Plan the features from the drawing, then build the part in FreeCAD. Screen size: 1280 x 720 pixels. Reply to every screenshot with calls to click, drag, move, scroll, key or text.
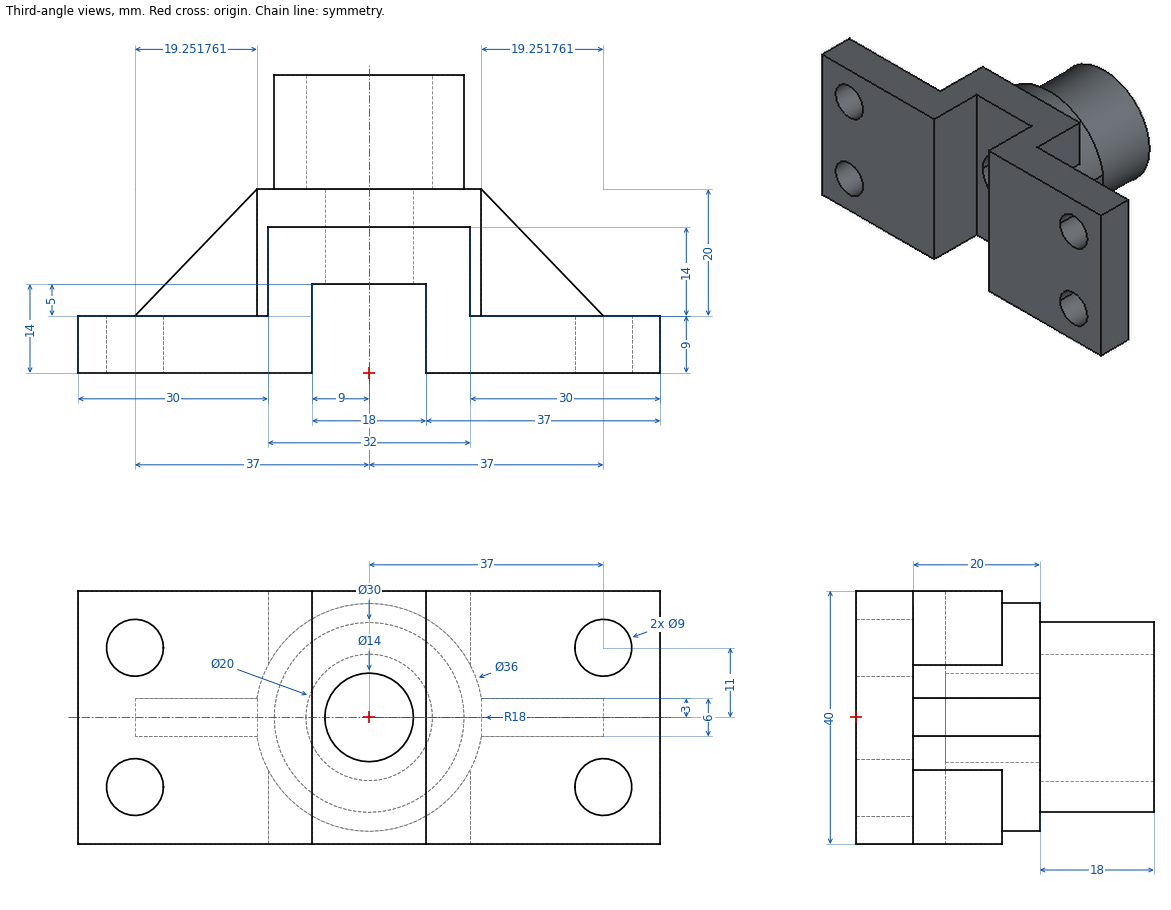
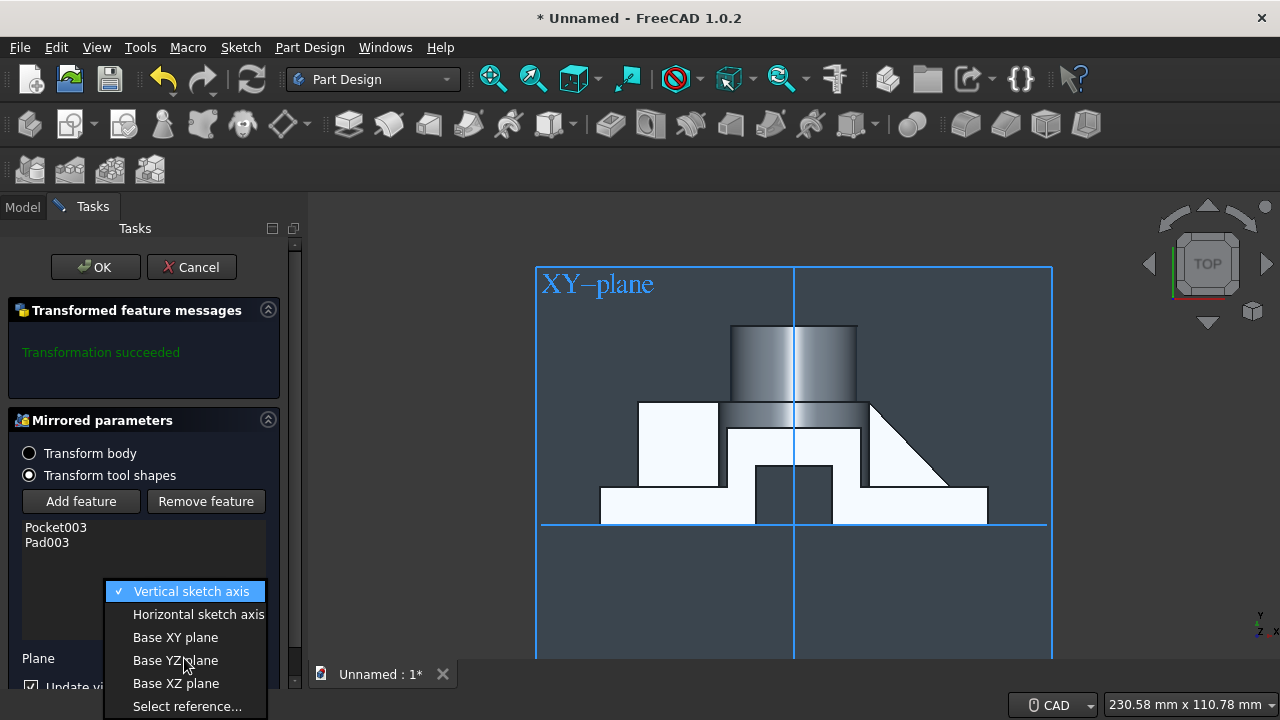
click(184, 660)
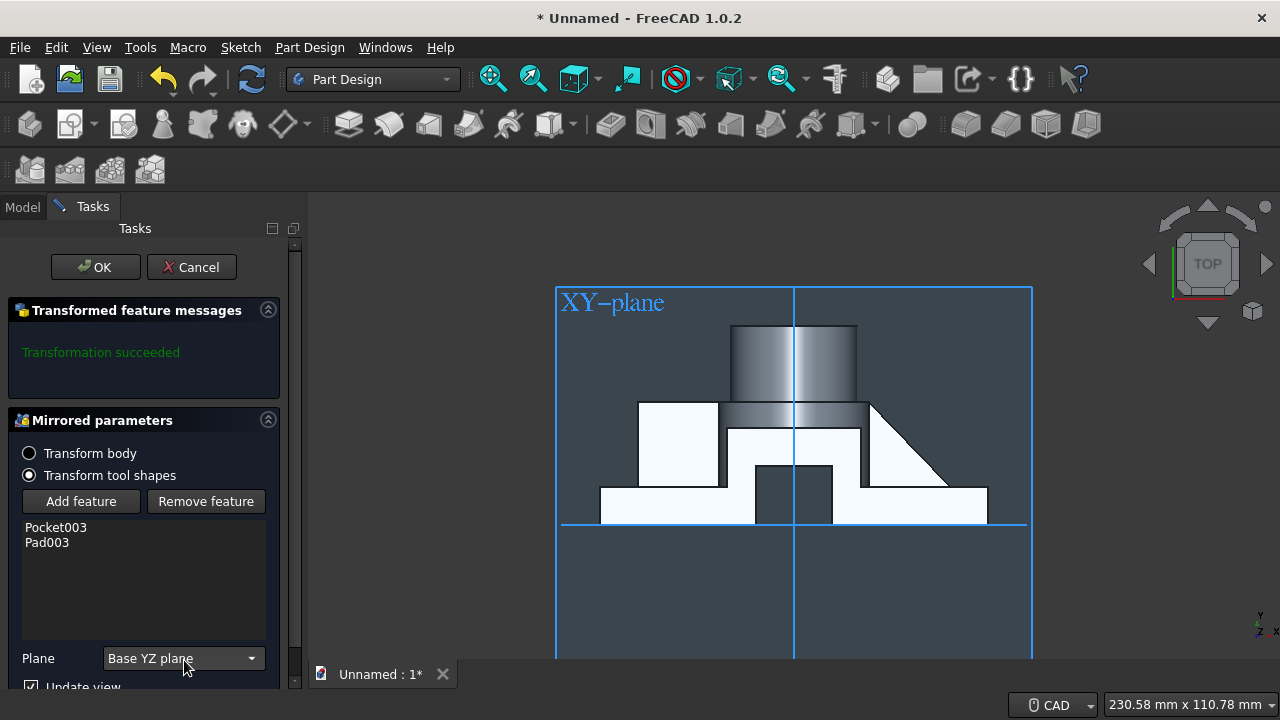
click(96, 267)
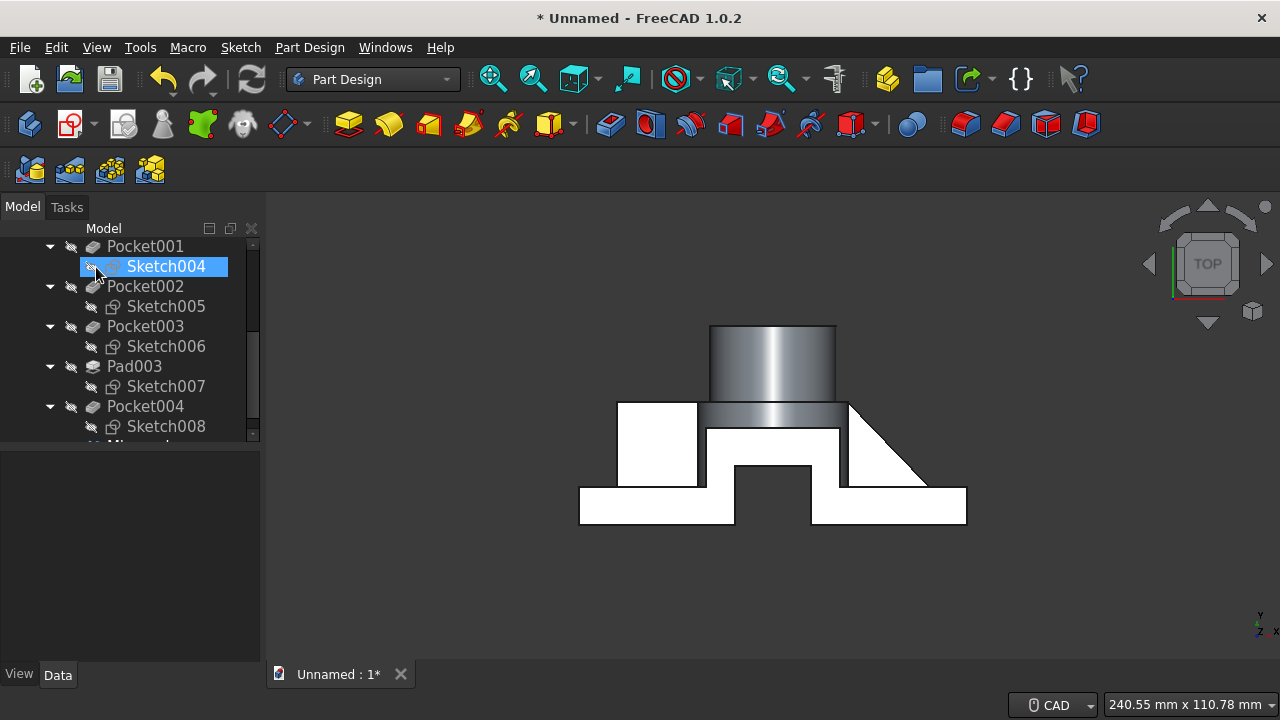
key(v)
key(f)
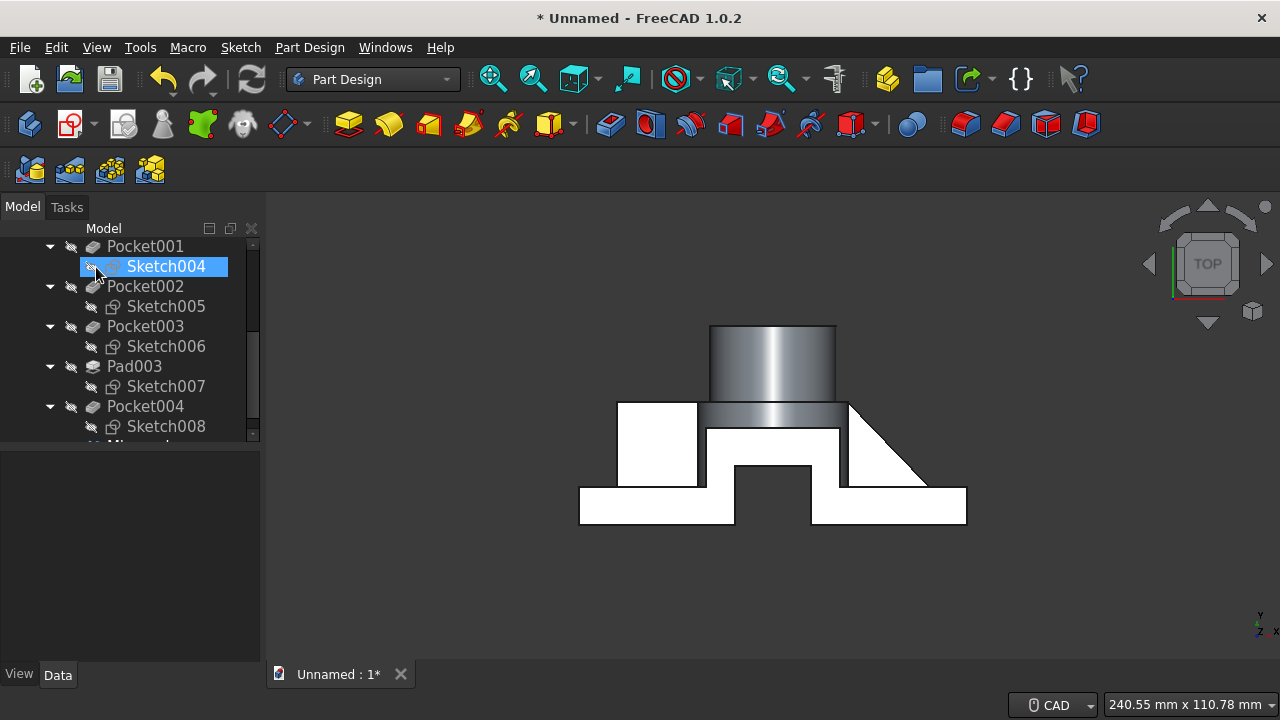
click(658, 443)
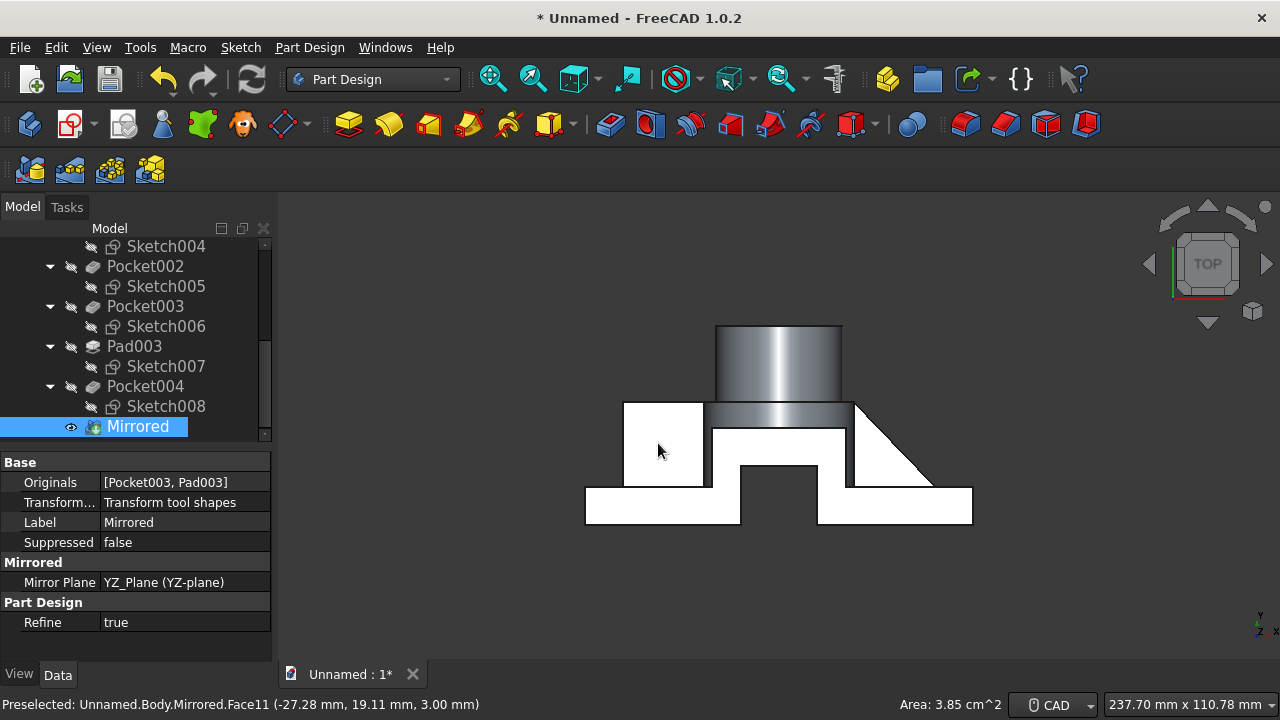
click(70, 124)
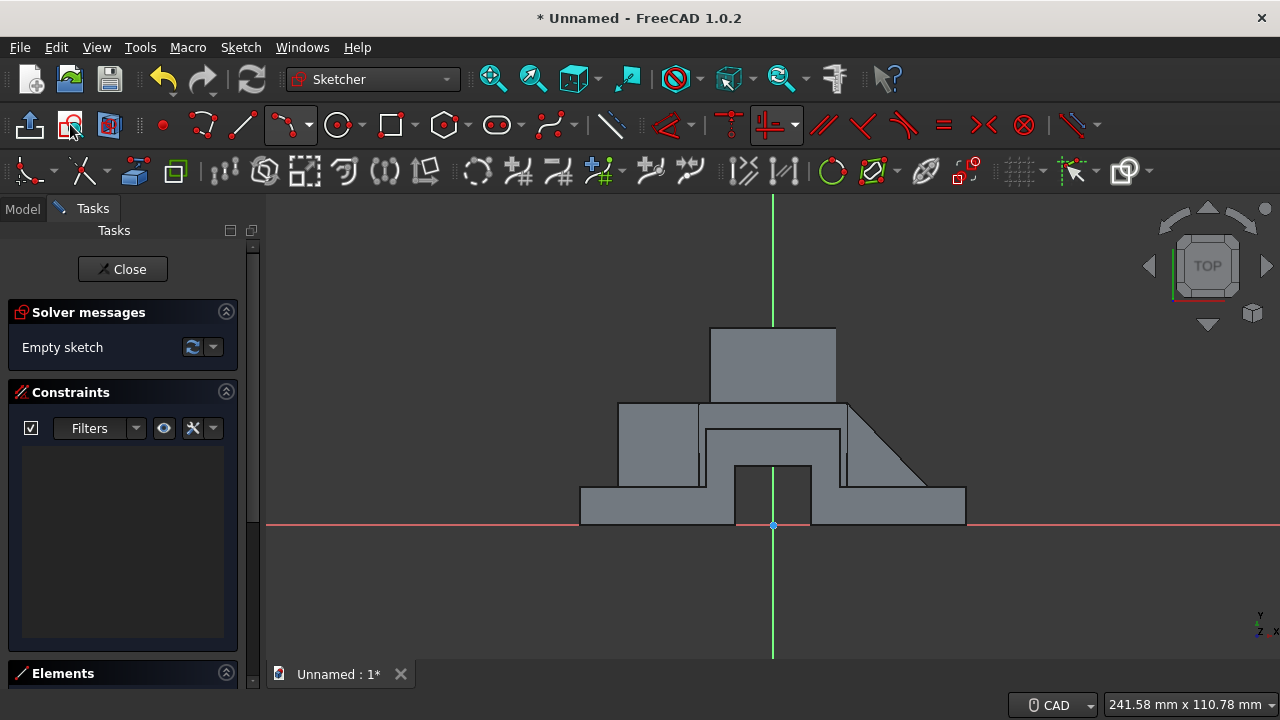
scroll(688, 495, up, 4)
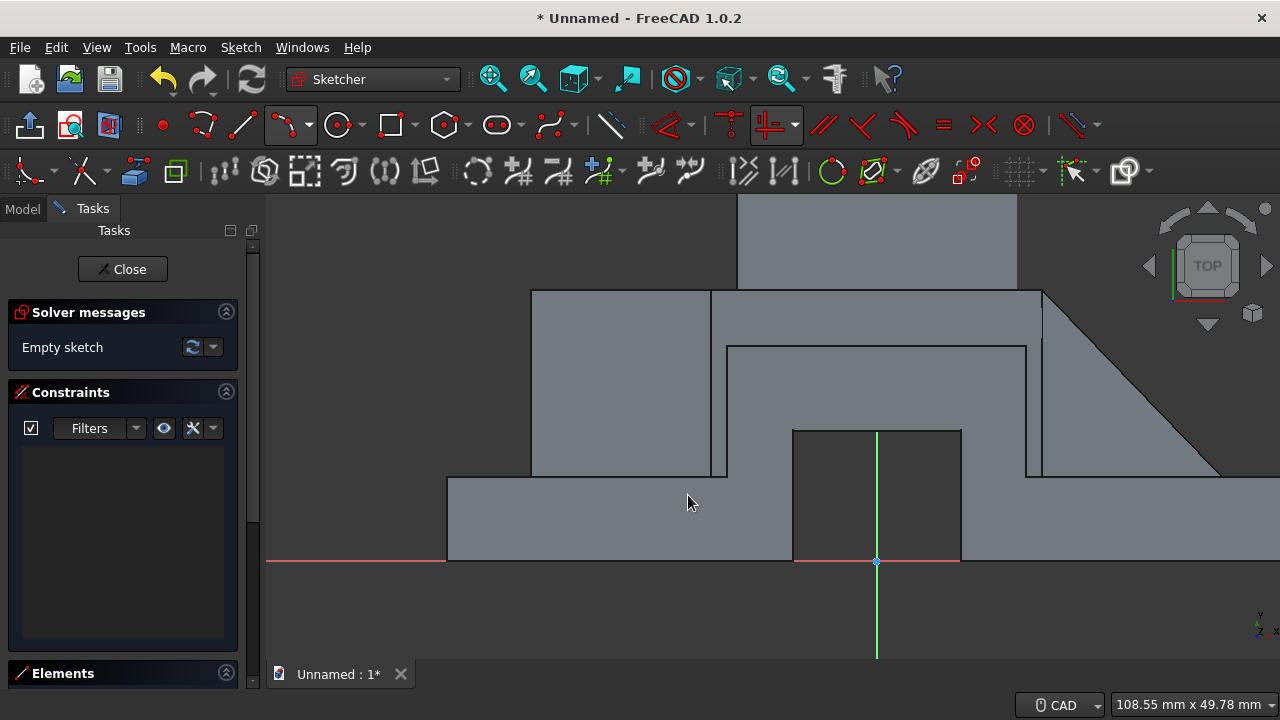
key(g)
key(m)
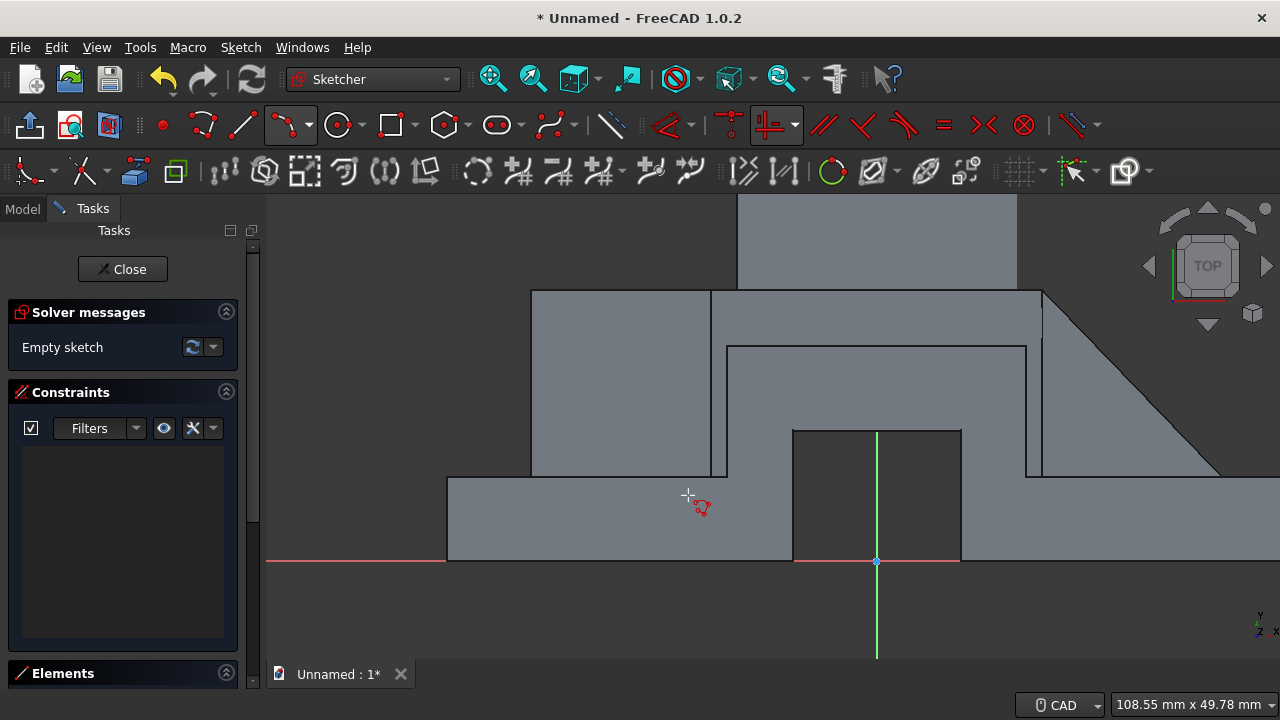
click(711, 290)
click(531, 290)
click(531, 477)
click(711, 291)
key(Escape)
key(Escape)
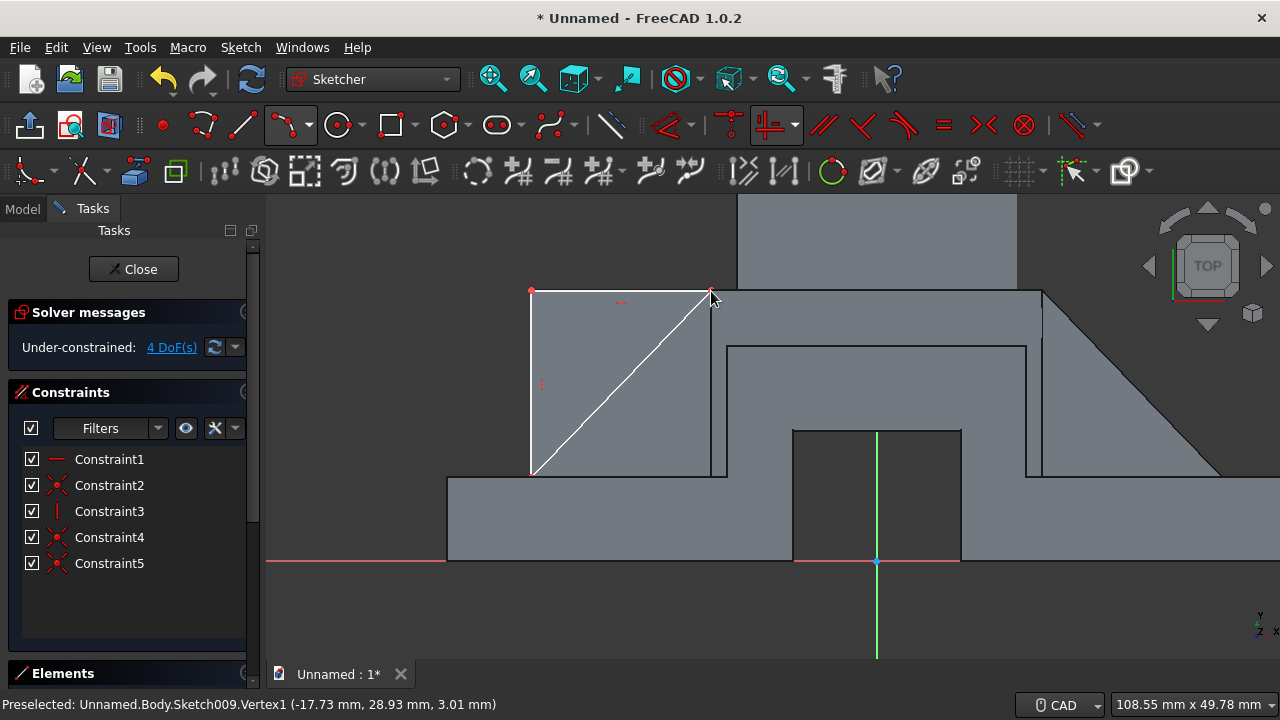
key(d)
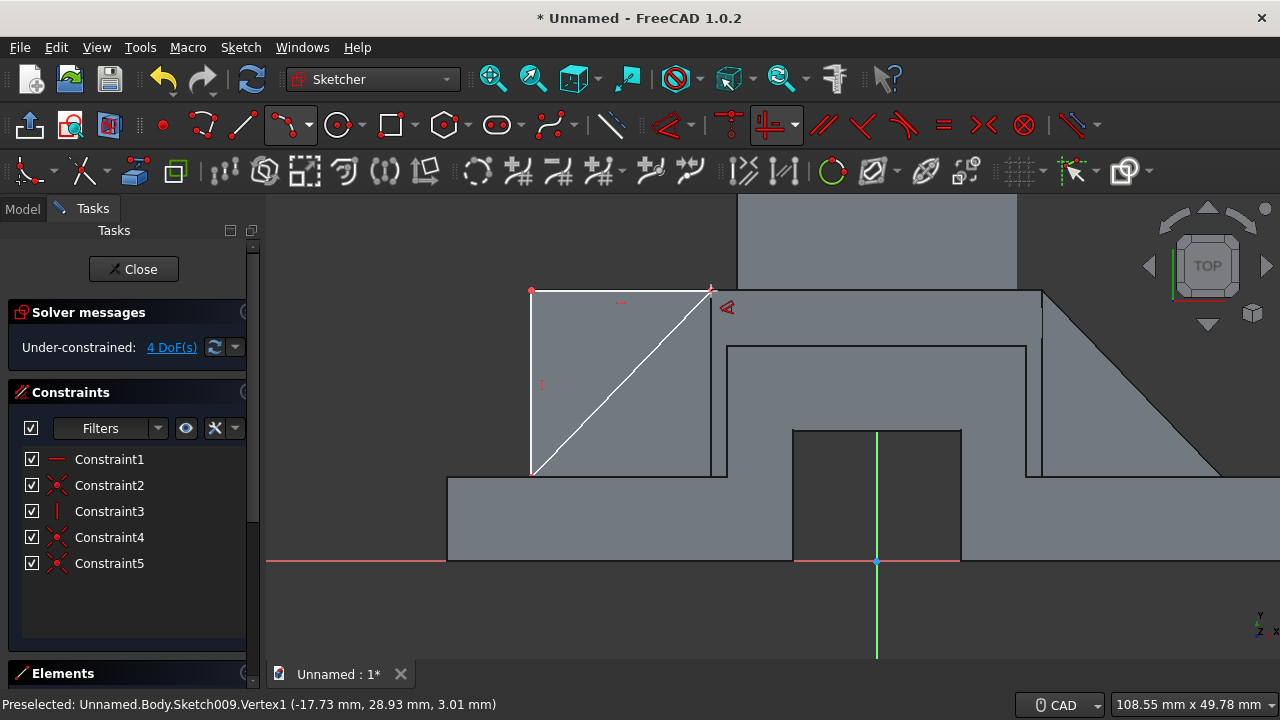
click(531, 347)
click(497, 384)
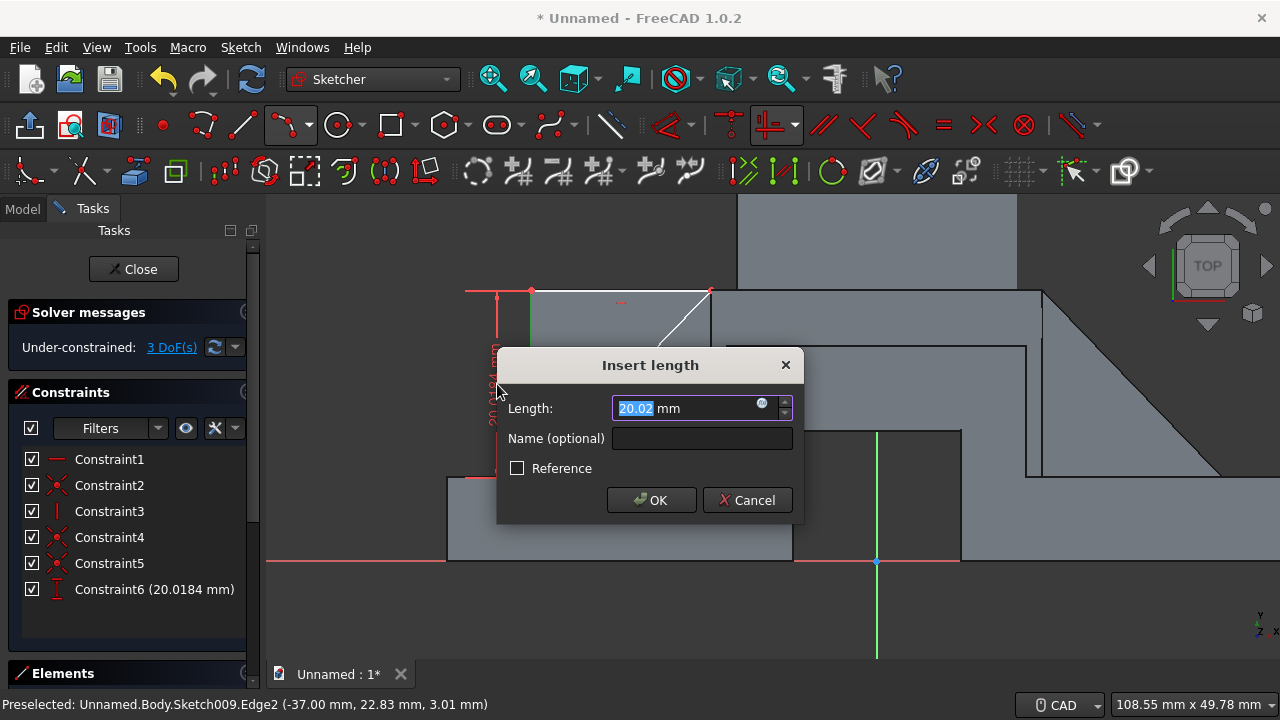
text(20)
key(Return)